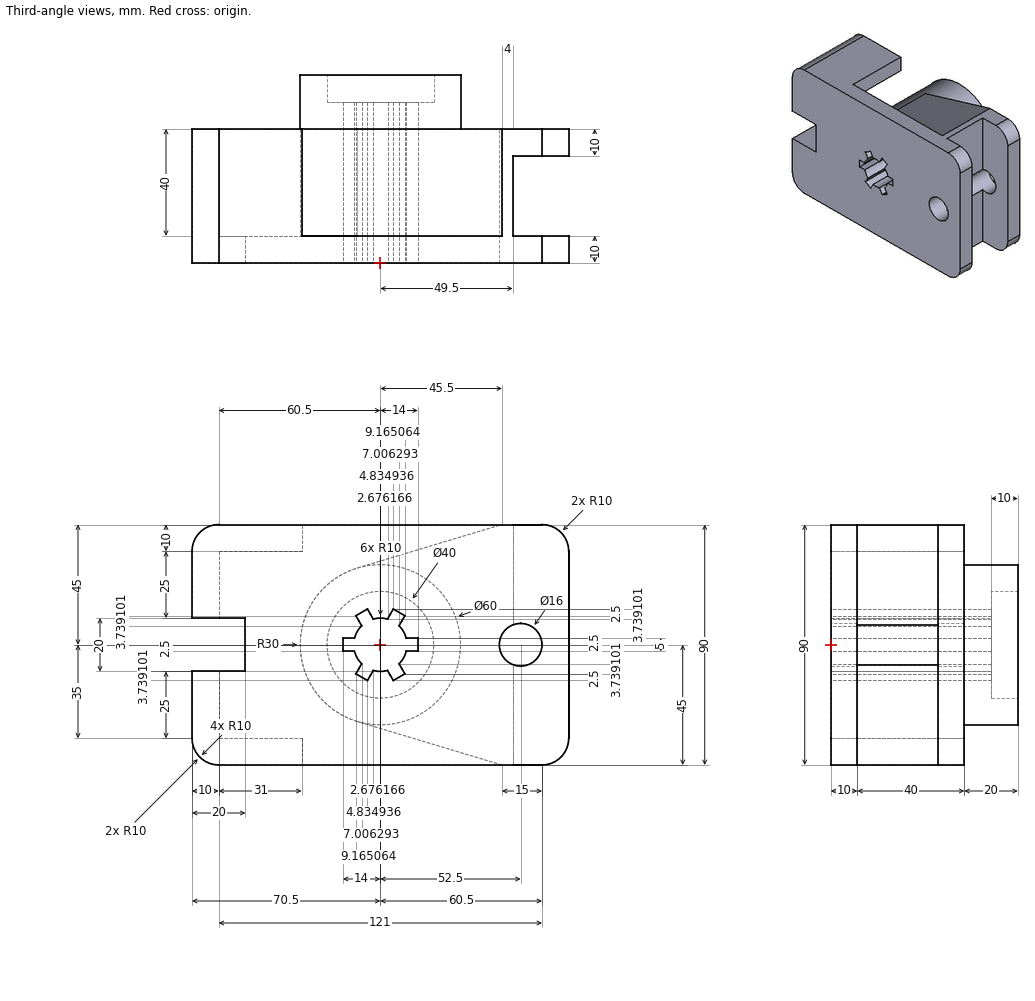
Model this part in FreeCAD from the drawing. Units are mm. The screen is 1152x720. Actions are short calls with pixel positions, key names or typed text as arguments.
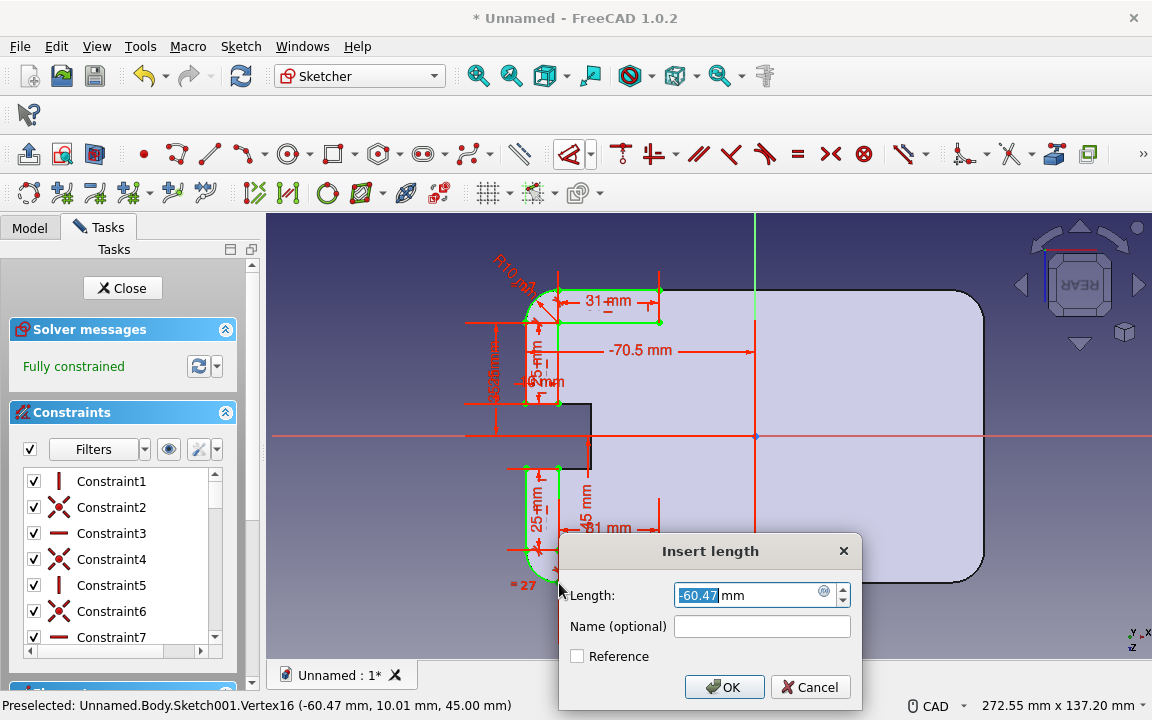
text(-60.5)
key(Return)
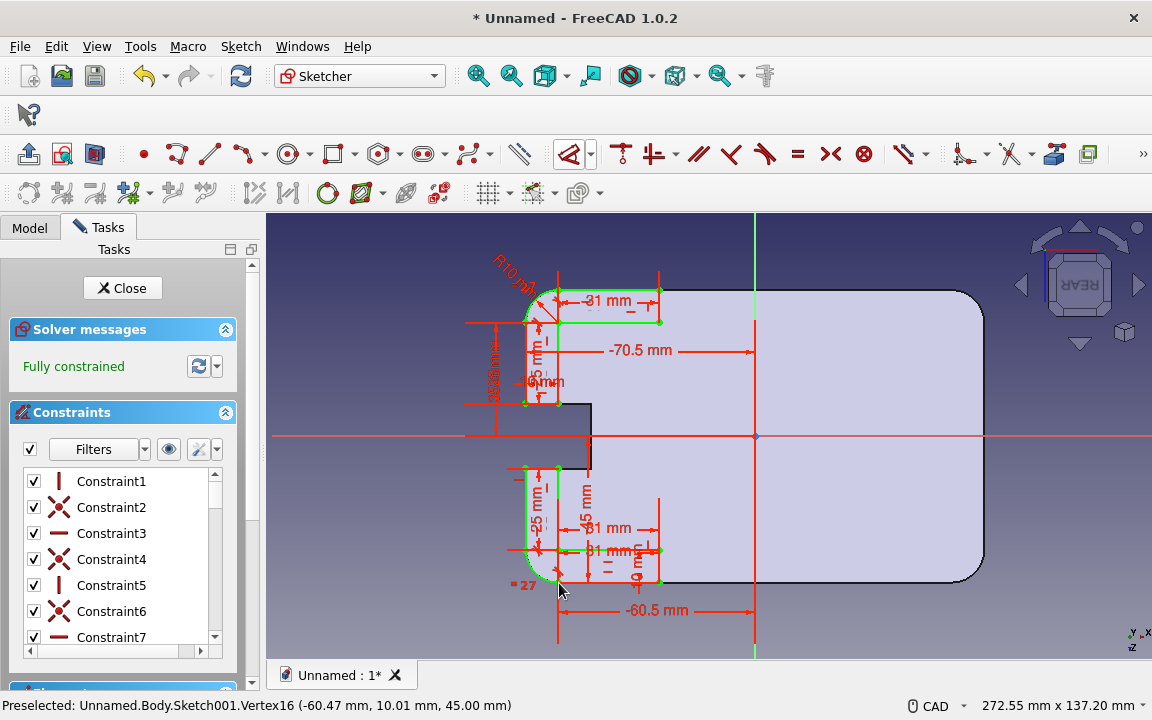
click(123, 288)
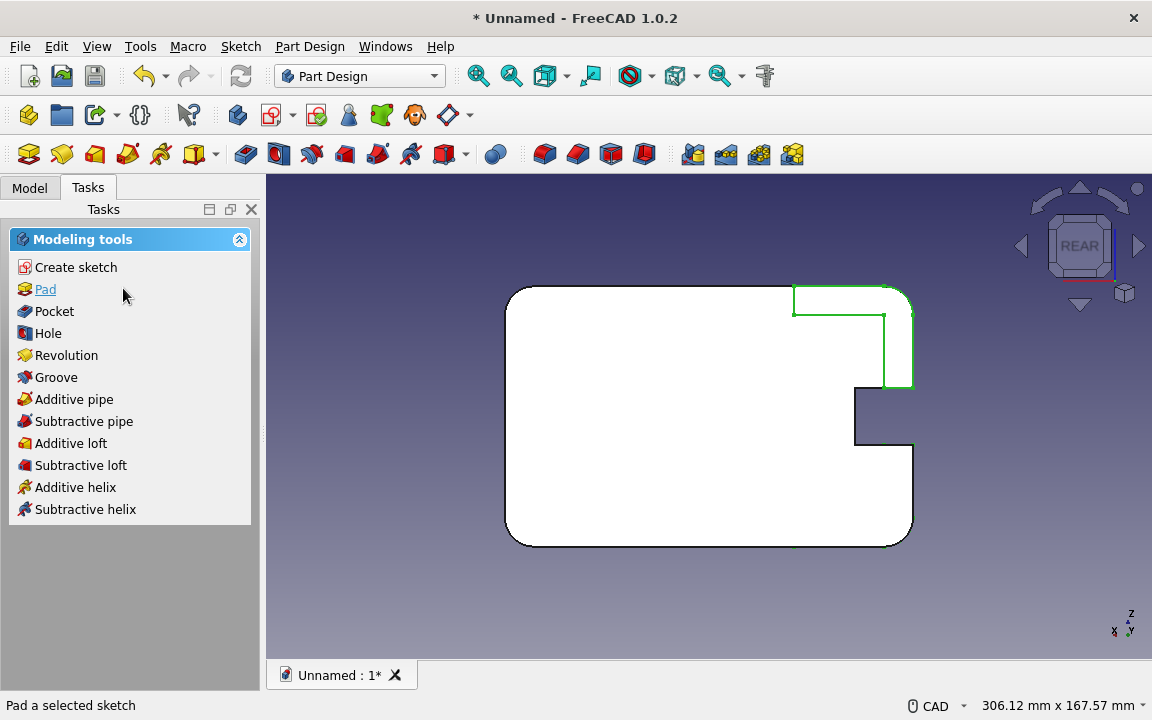
click(29, 154)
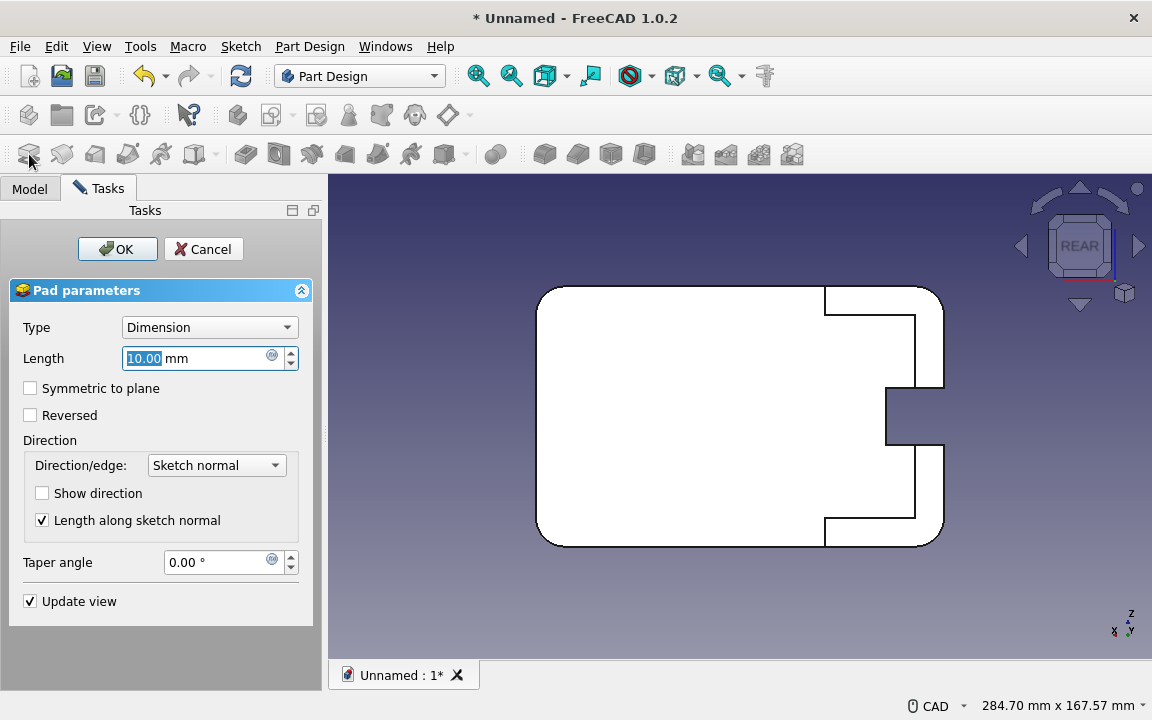
text(40)
key(Tab)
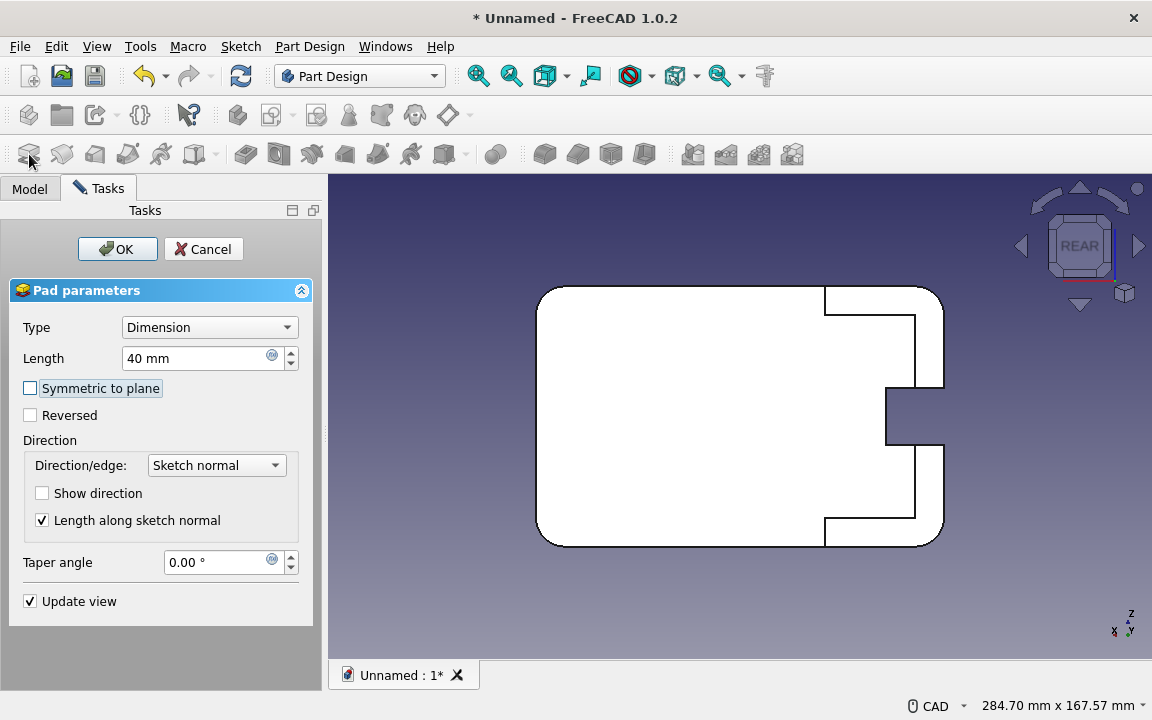
click(118, 249)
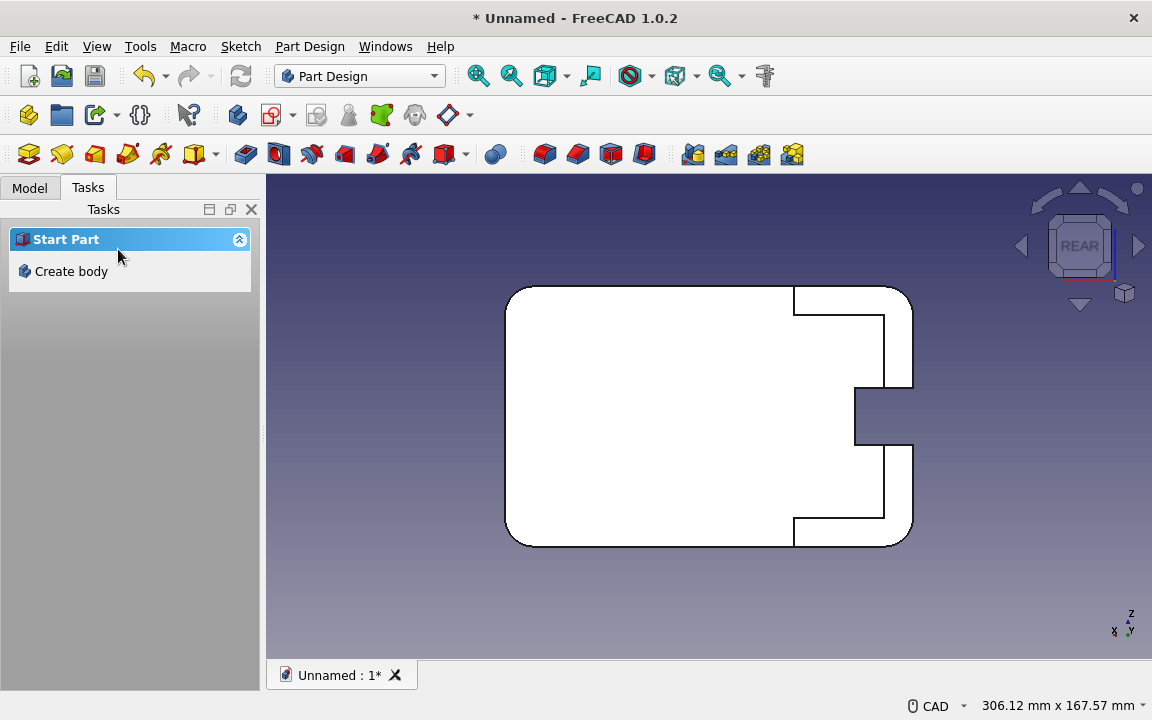
click(640, 416)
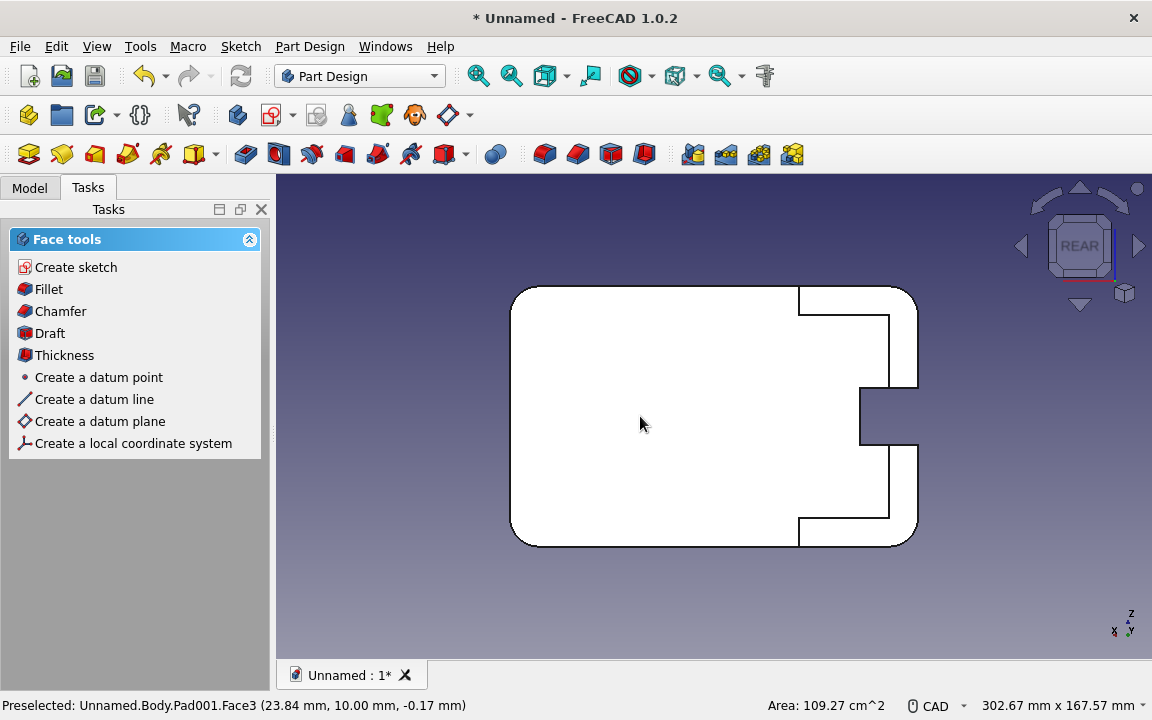
click(270, 116)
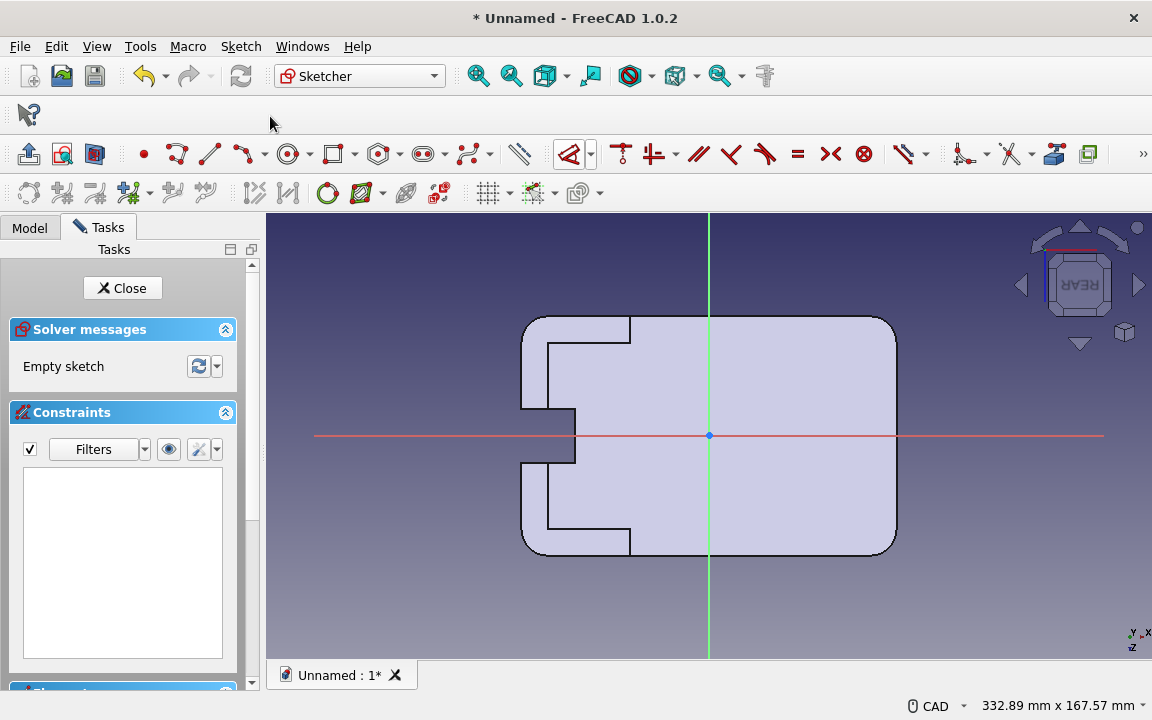
click(177, 154)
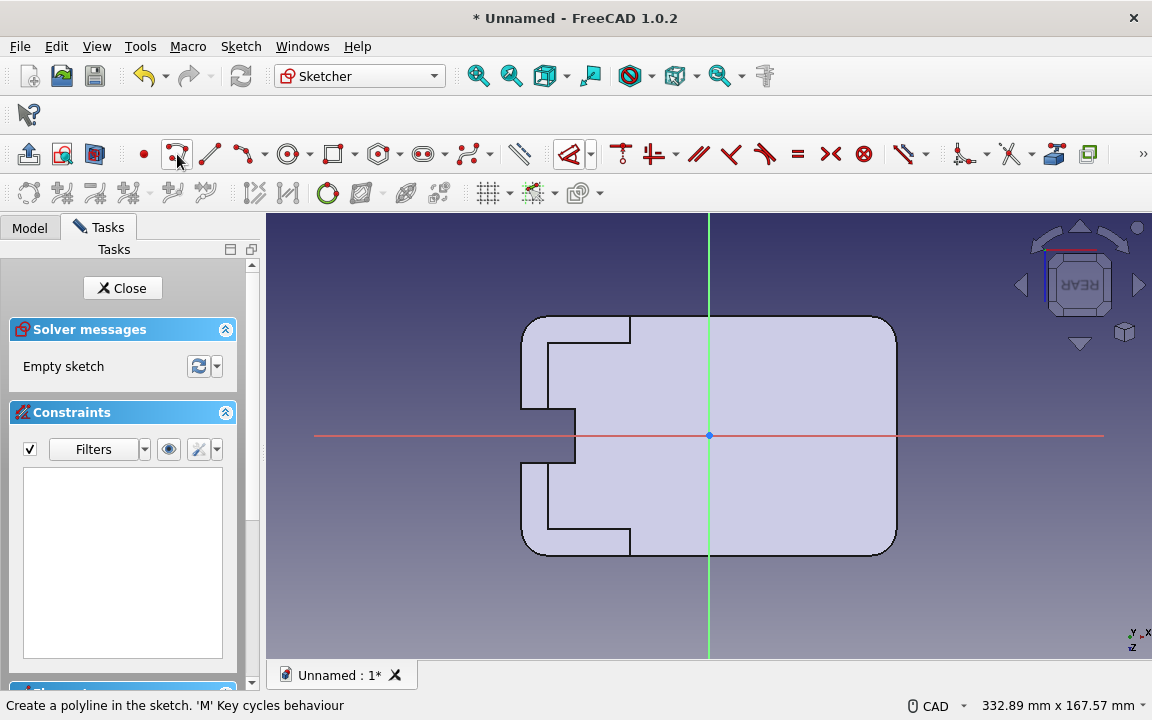
click(686, 512)
click(830, 556)
click(830, 316)
click(686, 360)
right_click(686, 360)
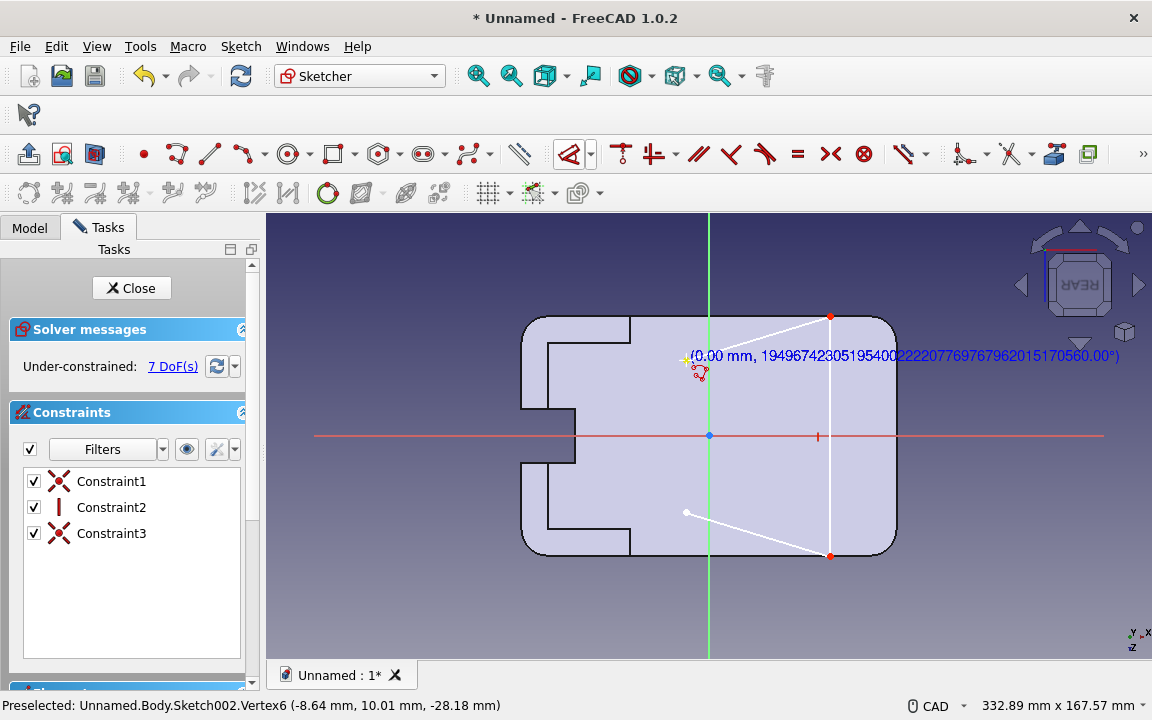
click(242, 154)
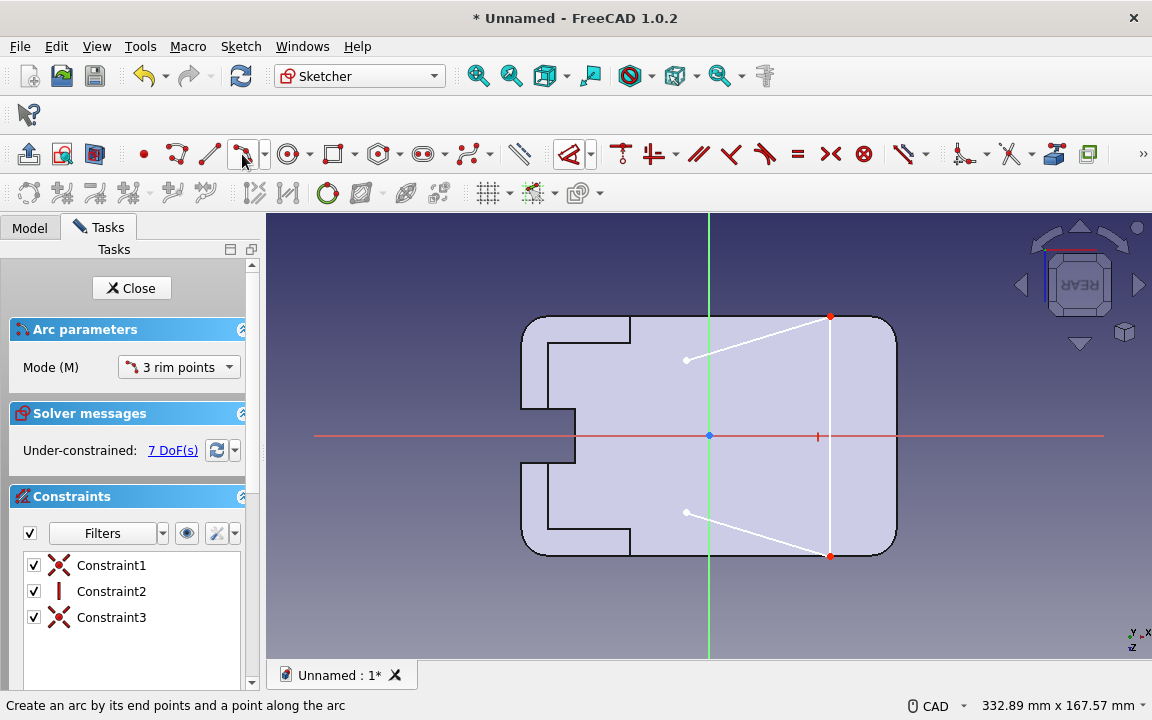
click(686, 361)
click(686, 513)
click(632, 416)
key(Escape)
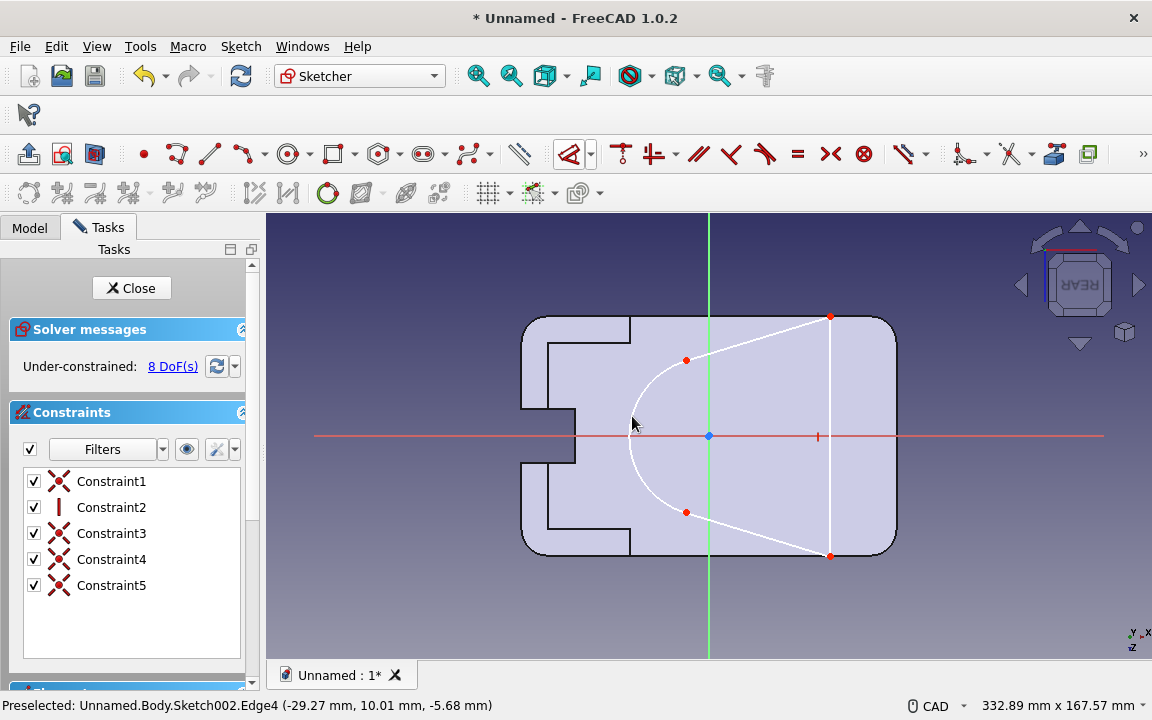
click(729, 526)